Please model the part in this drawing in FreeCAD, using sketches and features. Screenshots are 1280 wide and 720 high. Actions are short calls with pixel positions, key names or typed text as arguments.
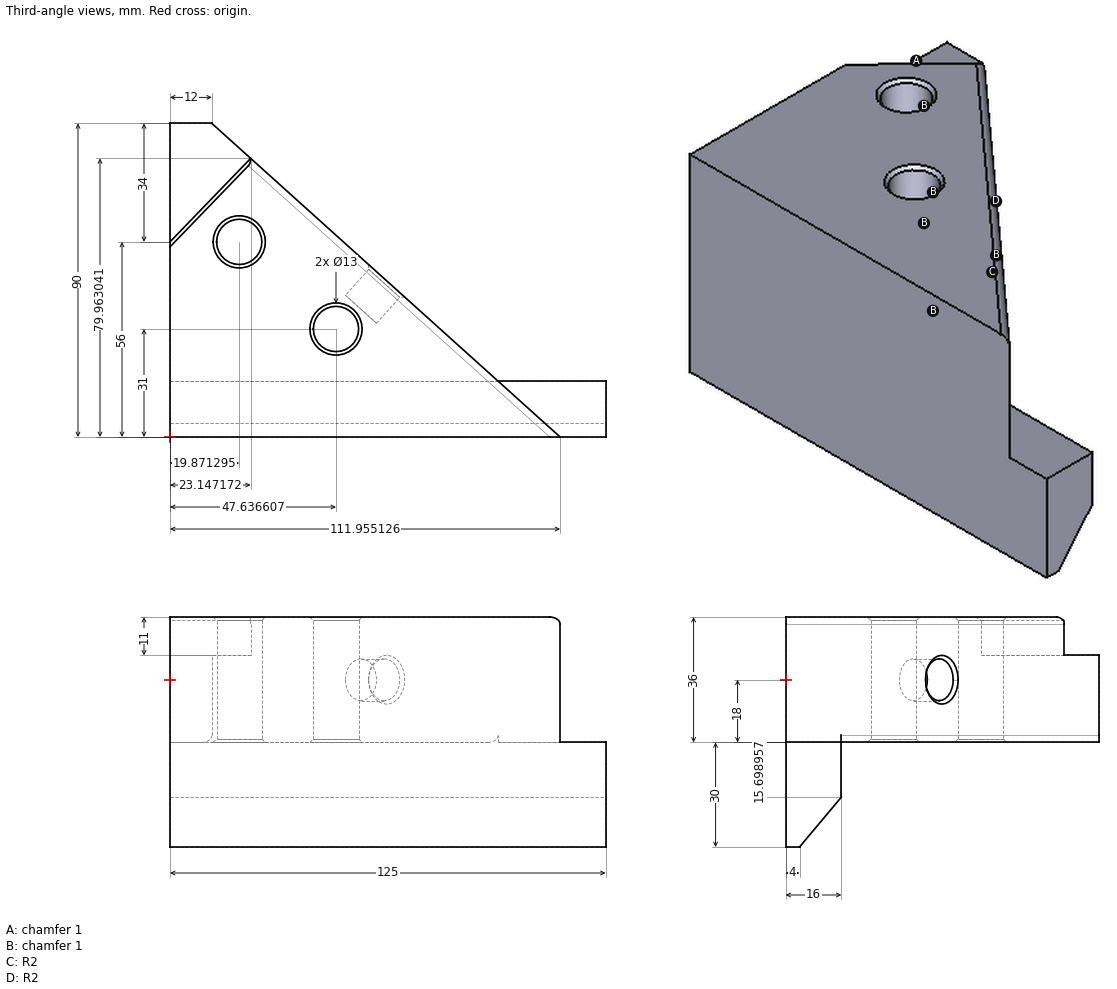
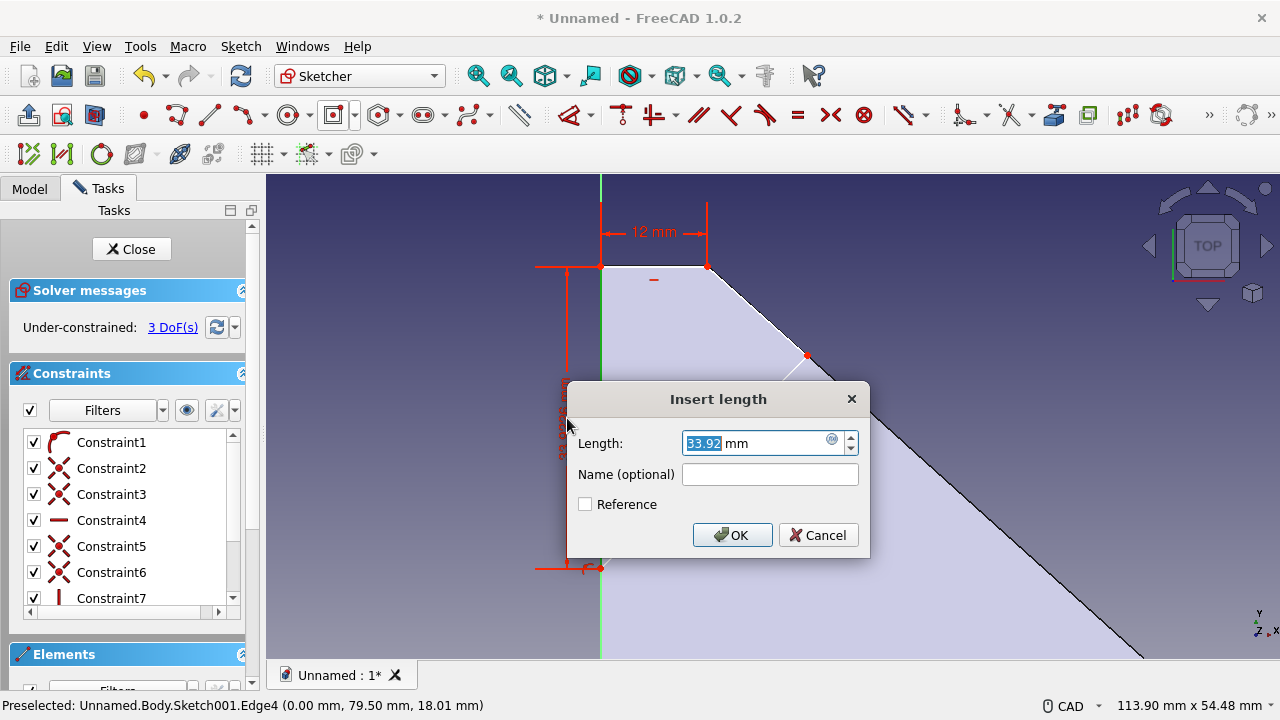
text(34)
key(Return)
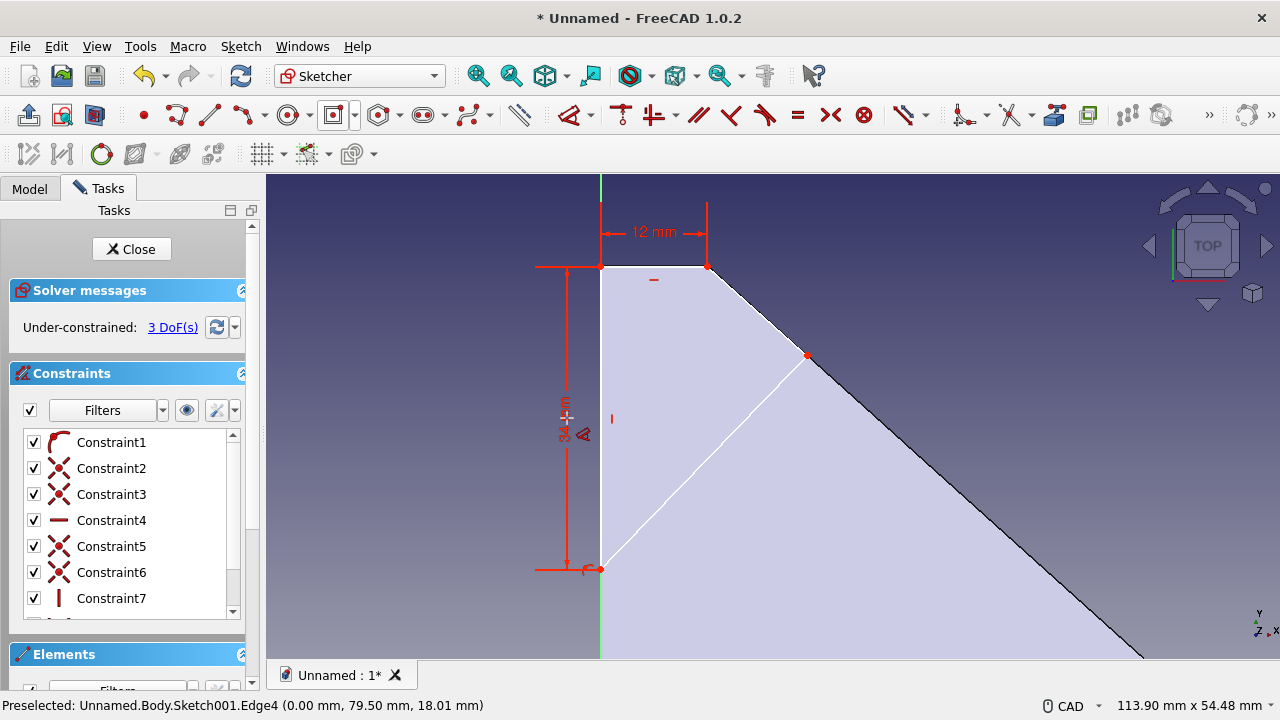
click(601, 570)
click(567, 600)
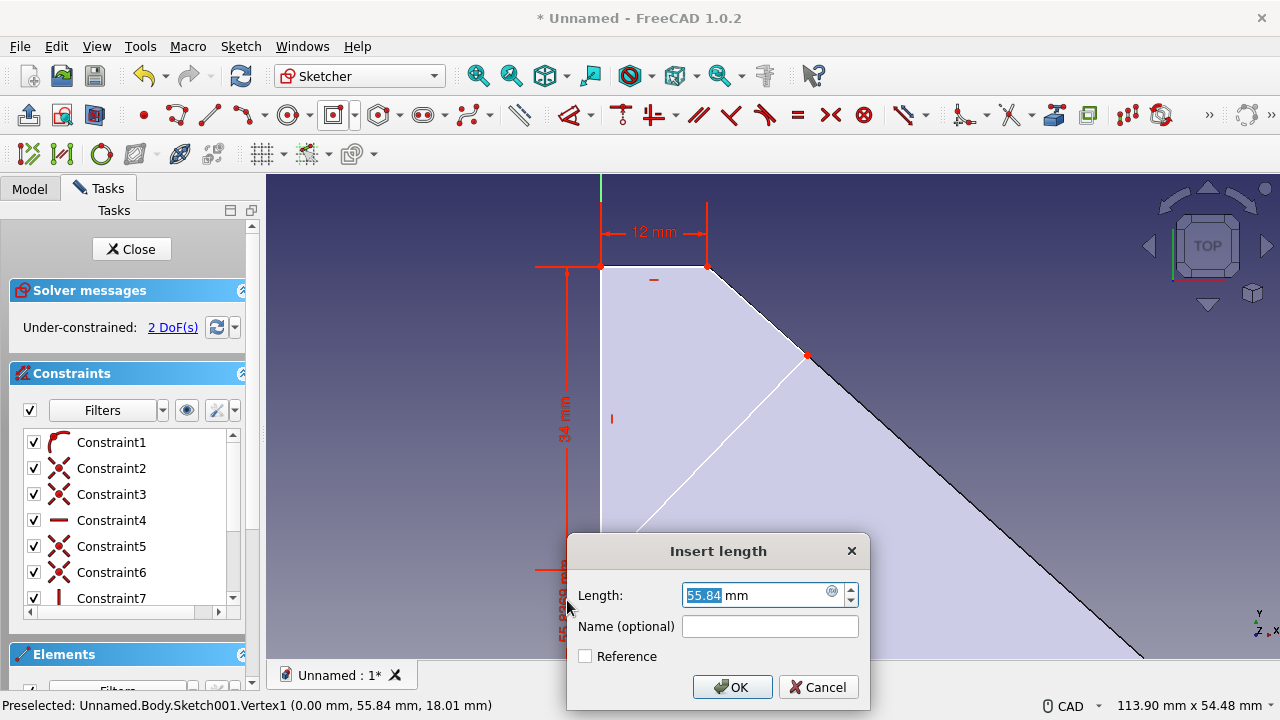
text(56)
key(Return)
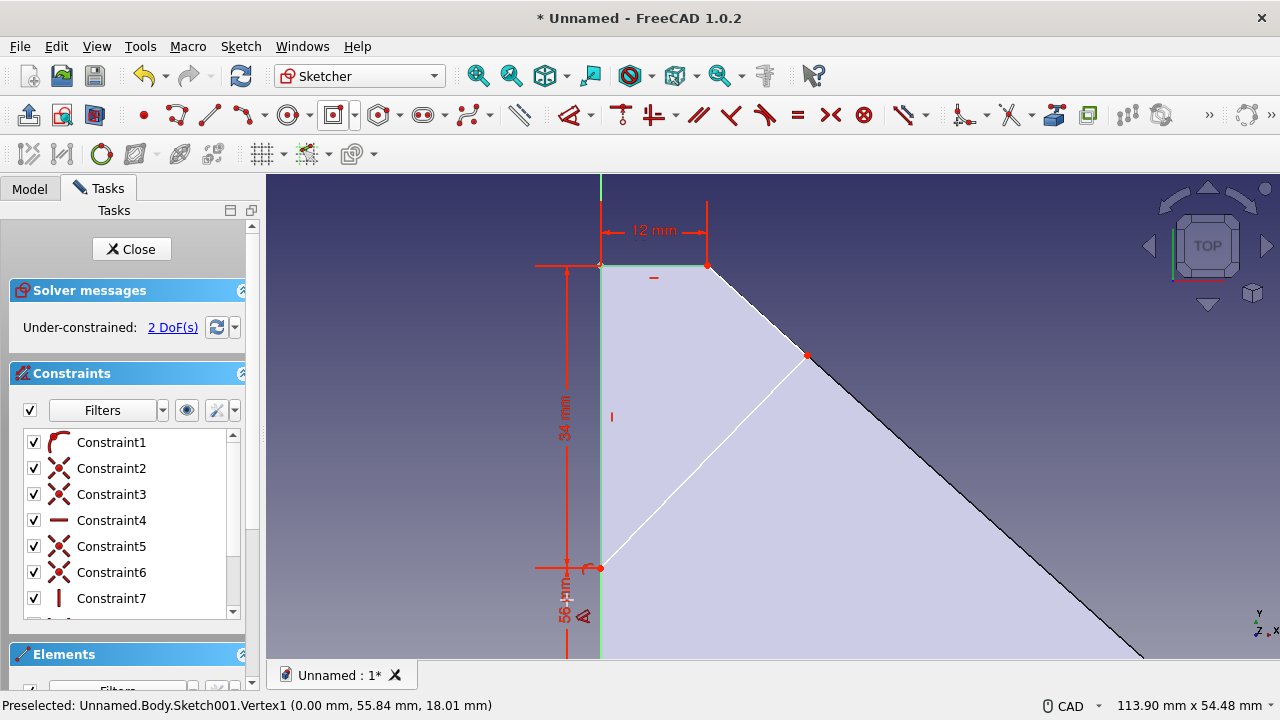
click(807, 356)
click(704, 322)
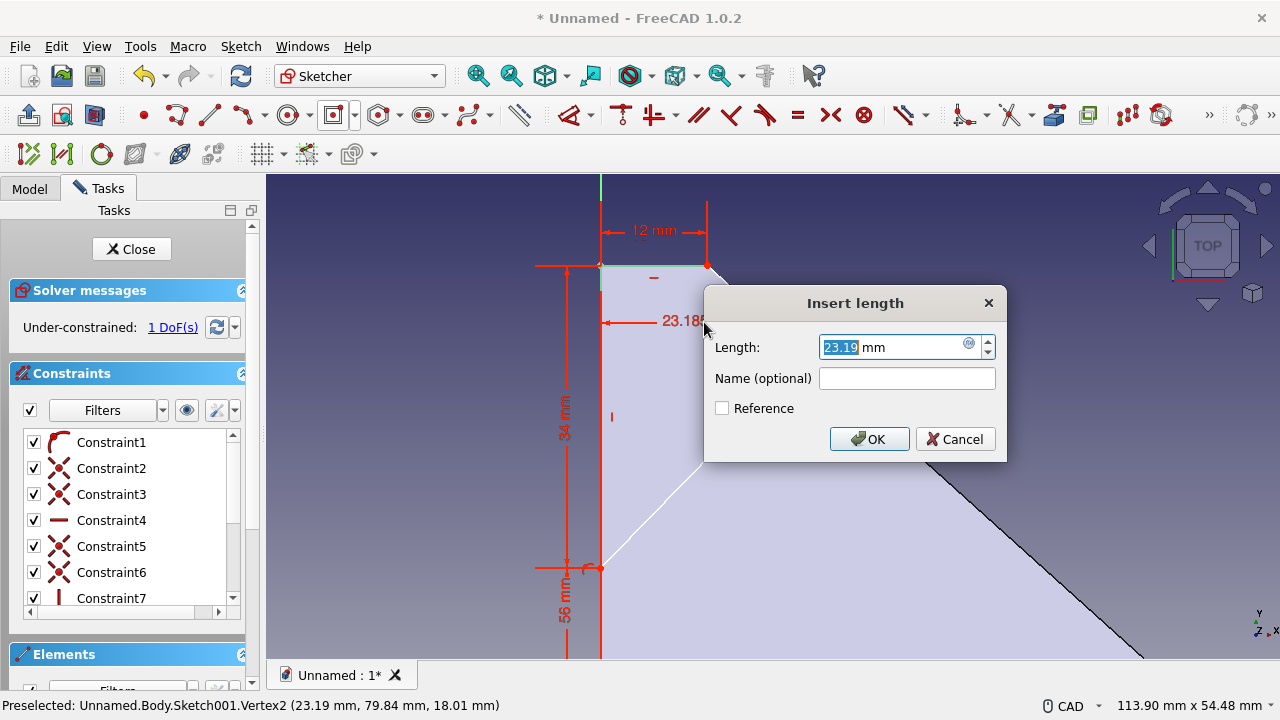
text(23.147172)
key(Return)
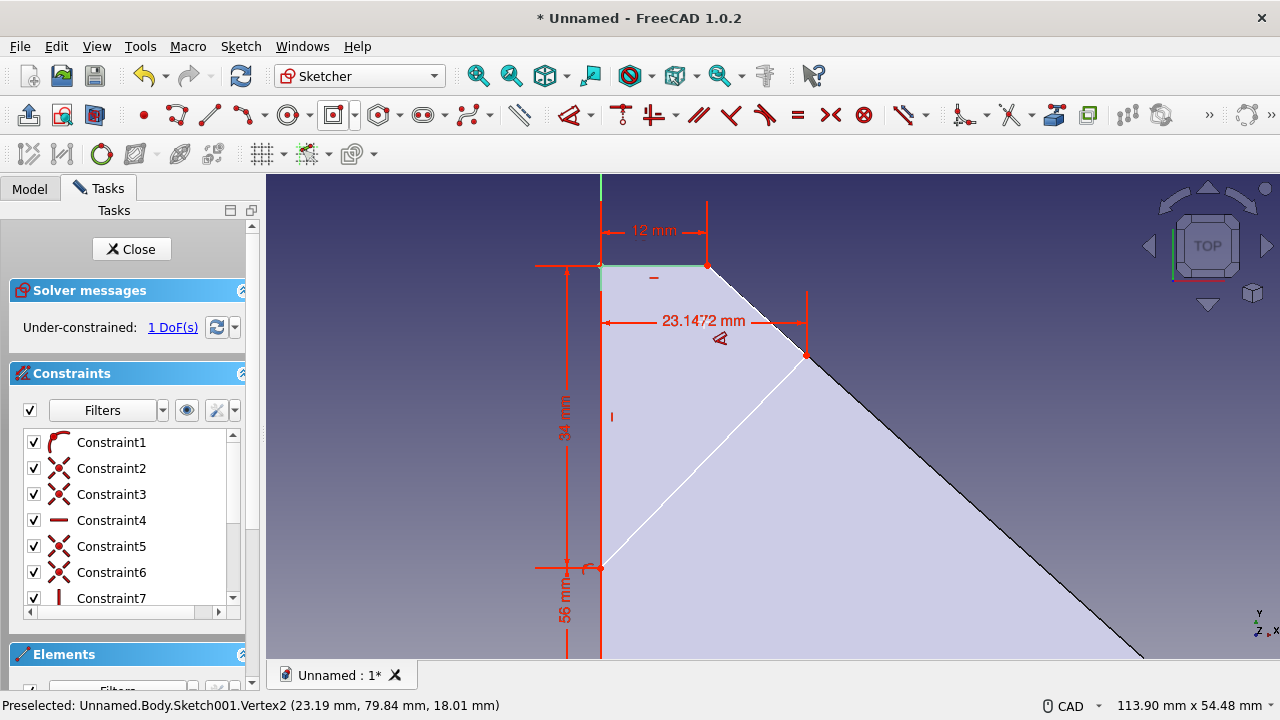
click(807, 356)
click(567, 493)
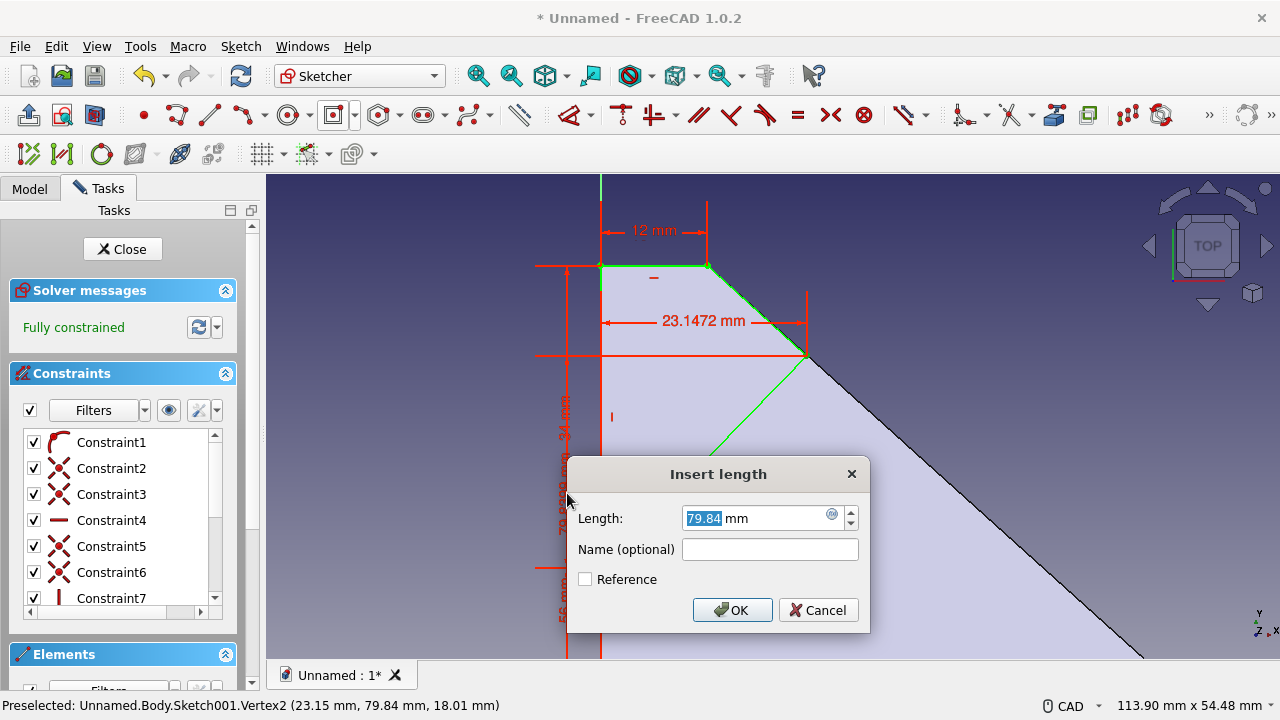
text(79.963041)
key(Return)
key(Escape)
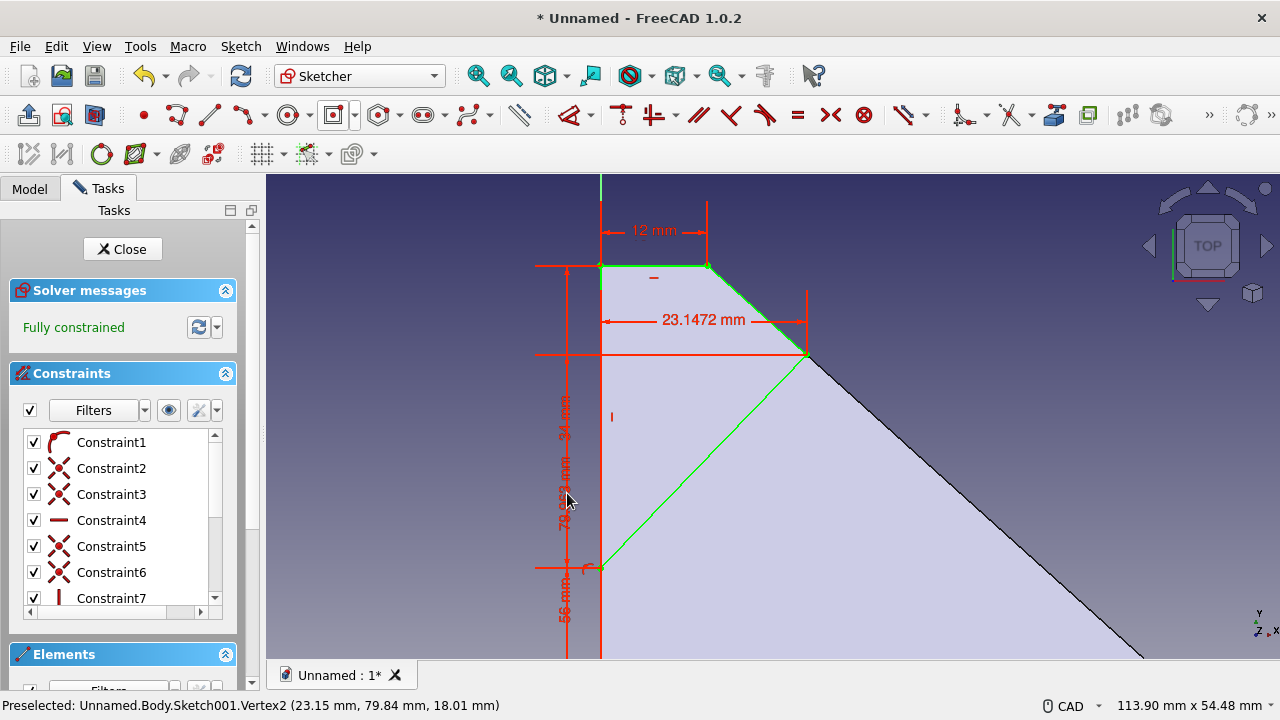
click(123, 249)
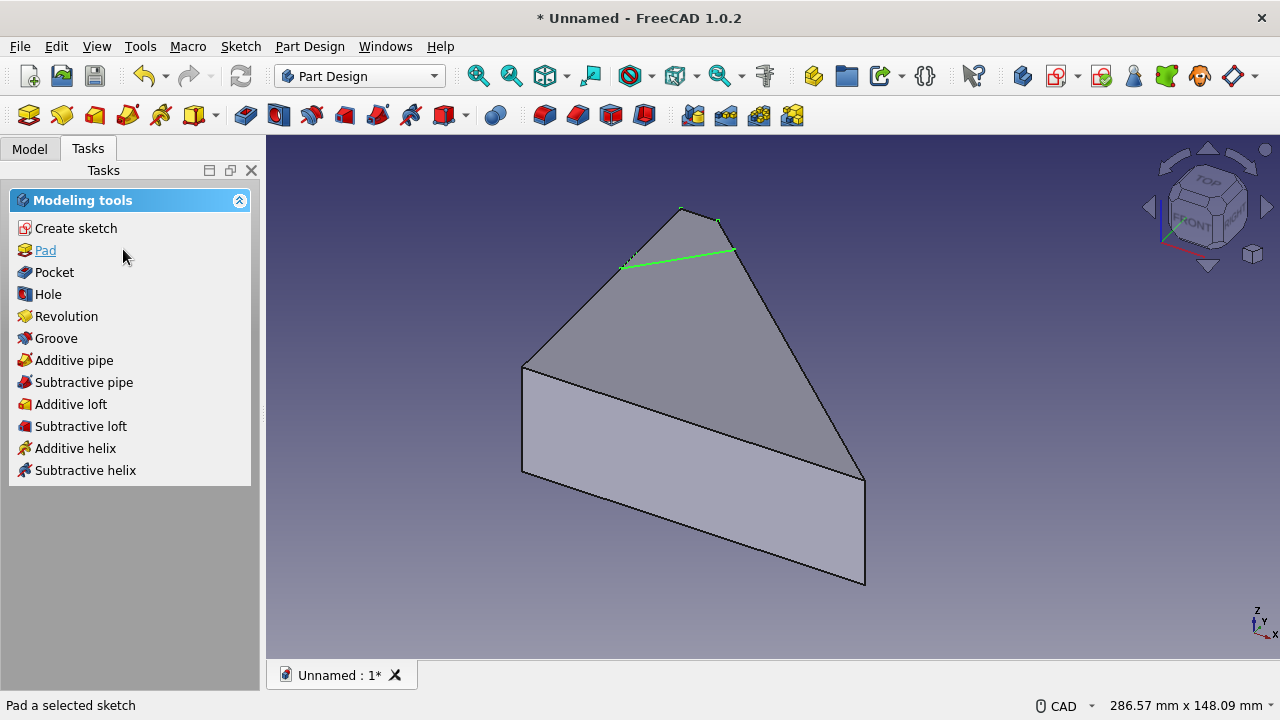
click(246, 116)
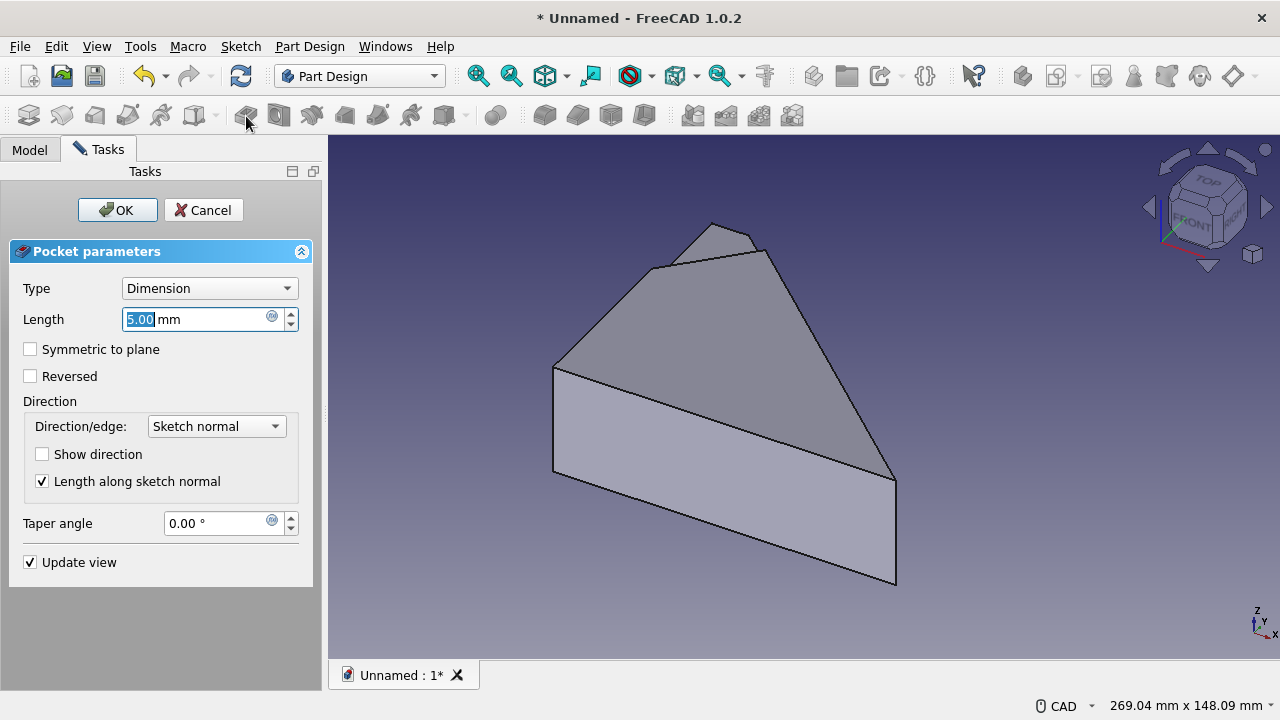
text(11)
key(Tab)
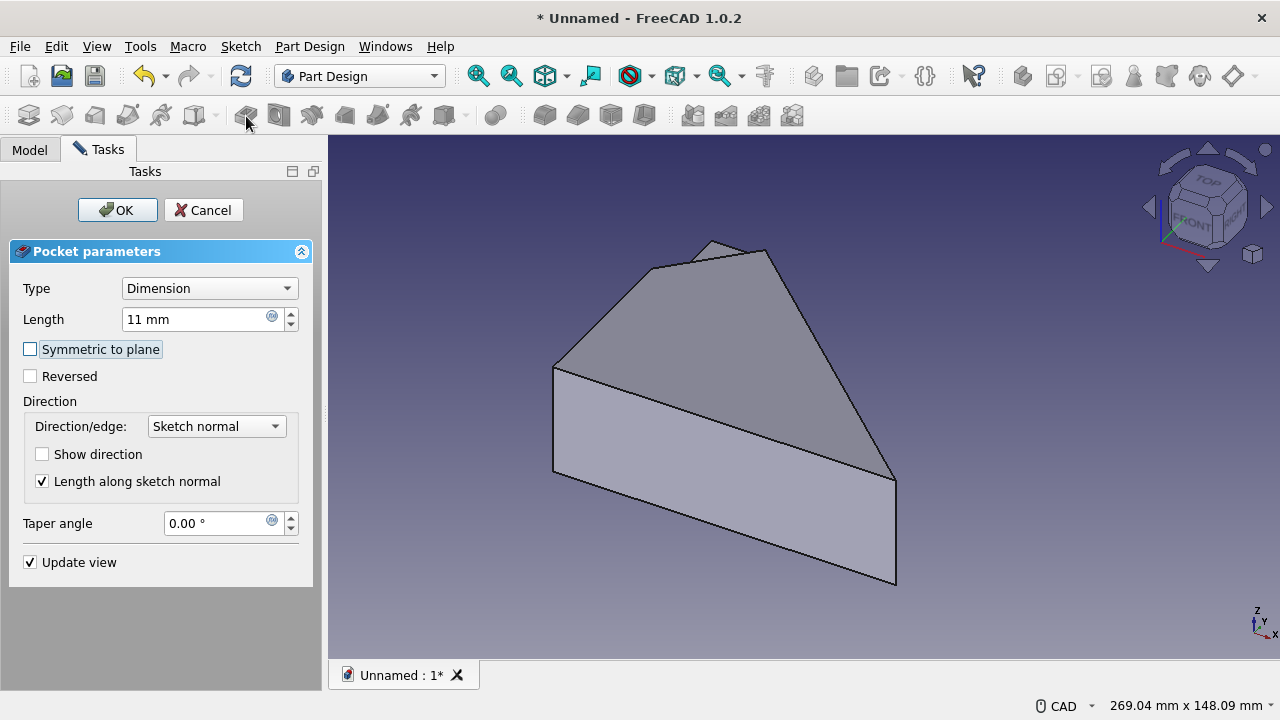
click(118, 210)